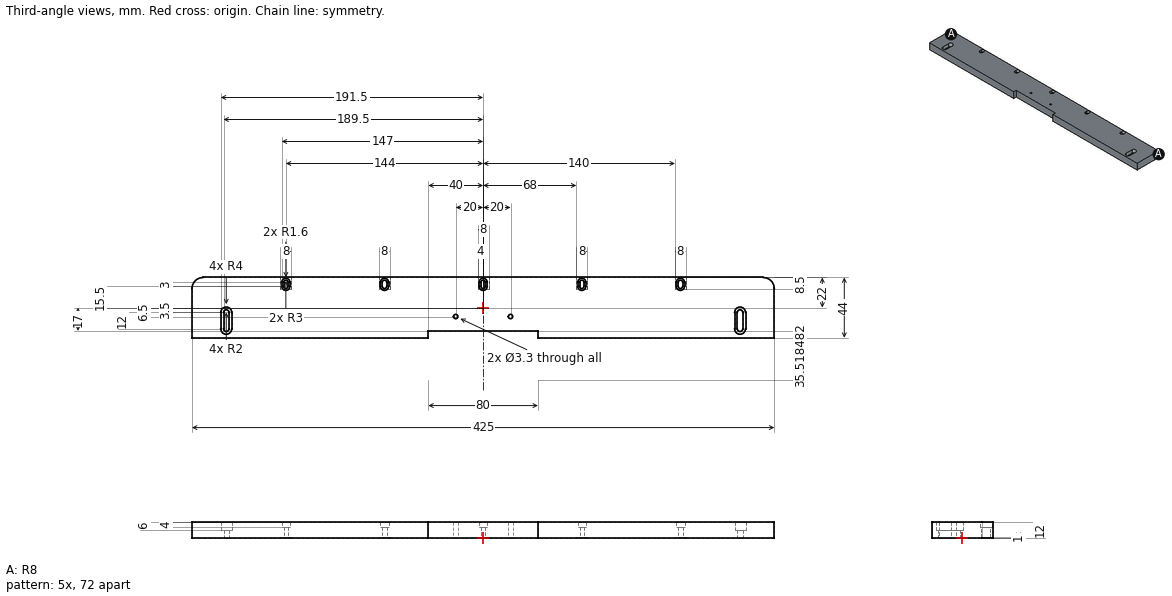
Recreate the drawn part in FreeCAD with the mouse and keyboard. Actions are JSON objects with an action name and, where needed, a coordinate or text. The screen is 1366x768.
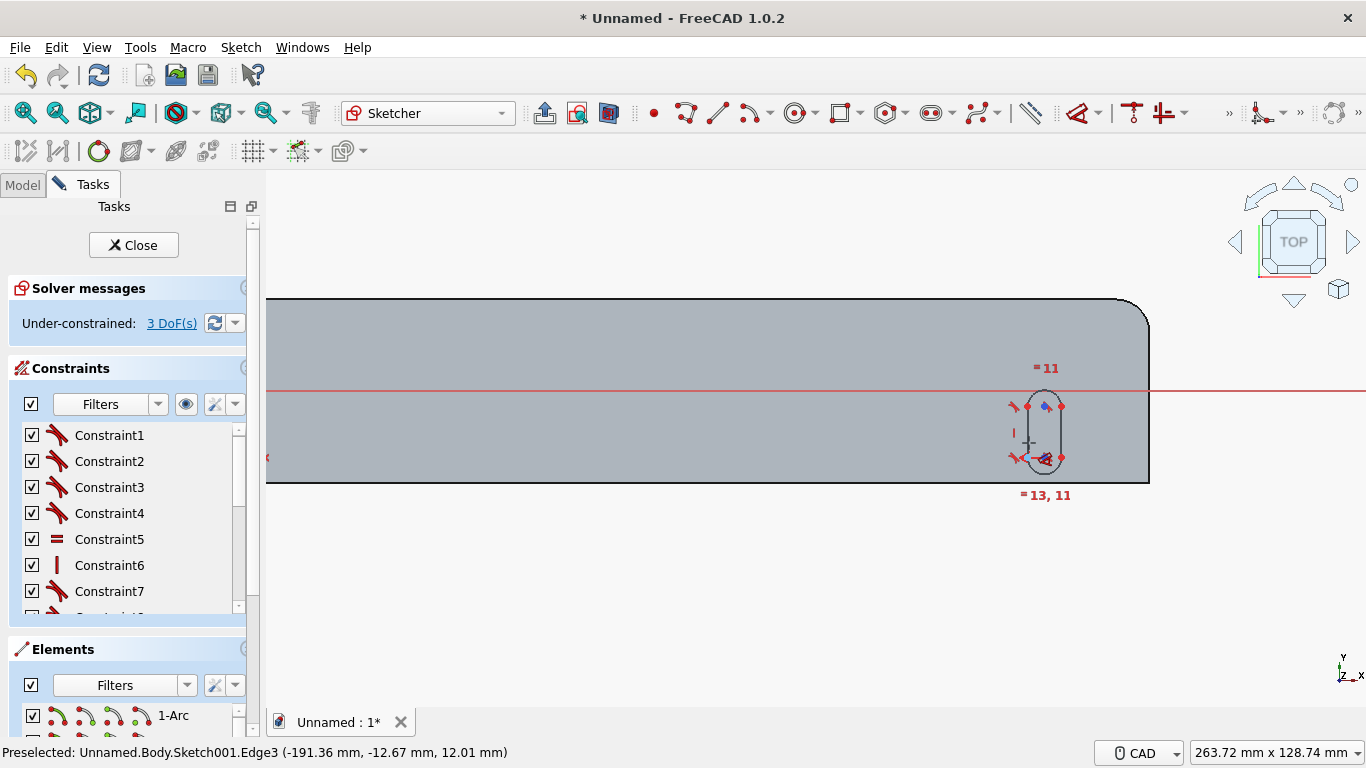
{"action": "left_click", "coordinate": [1028, 443]}
{"action": "left_click", "coordinate": [994, 432]}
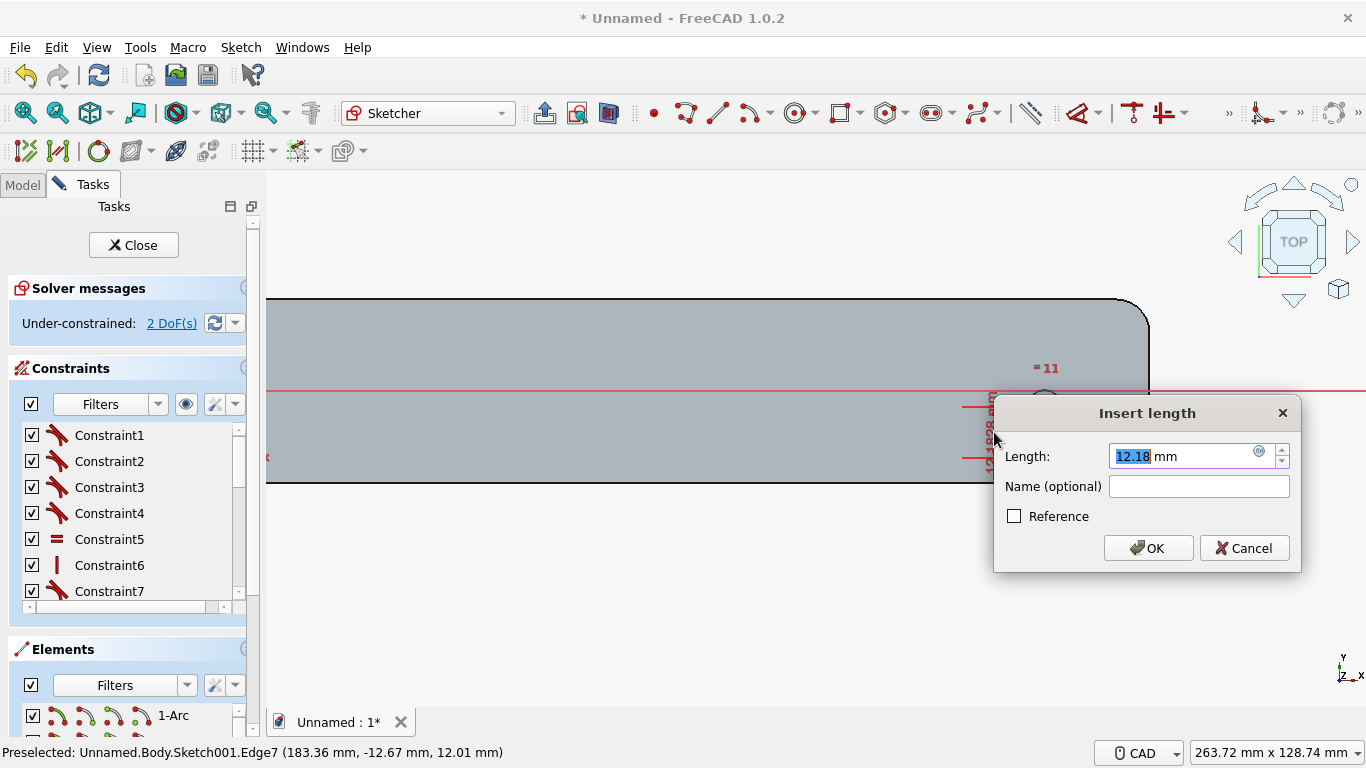
{"action": "type", "text": "12"}
{"action": "key", "text": "Return"}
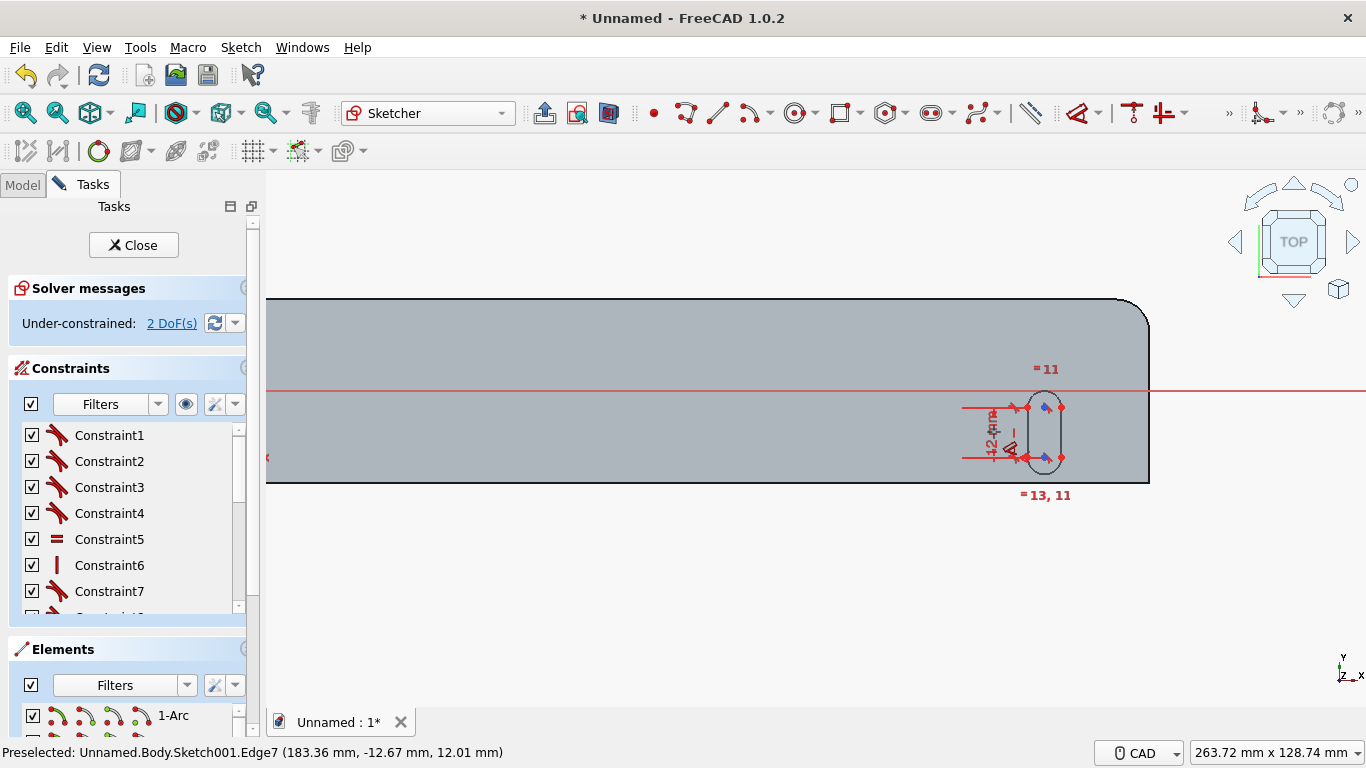
{"action": "scroll", "coordinate": [1029, 443], "scroll_direction": "down", "scroll_amount": 5}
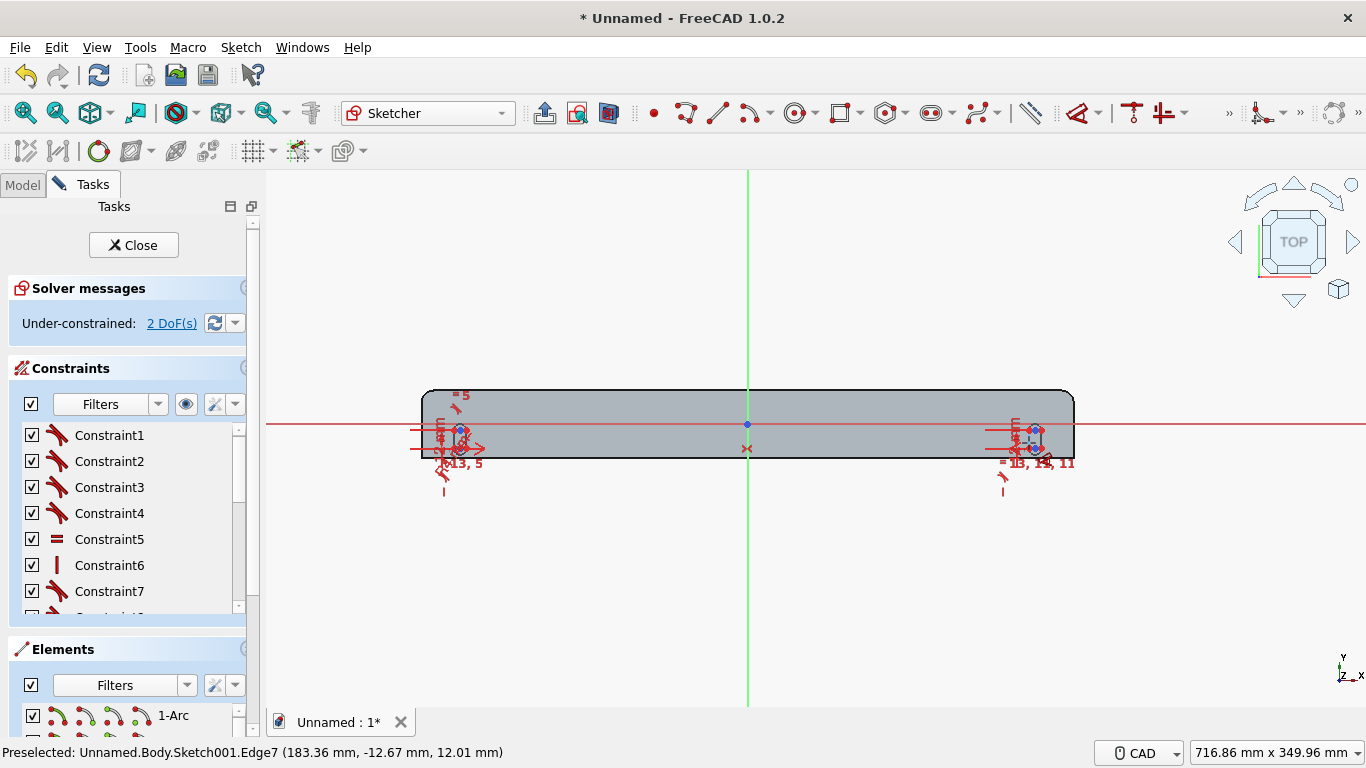
{"action": "scroll", "coordinate": [466, 430], "scroll_direction": "up", "scroll_amount": 11}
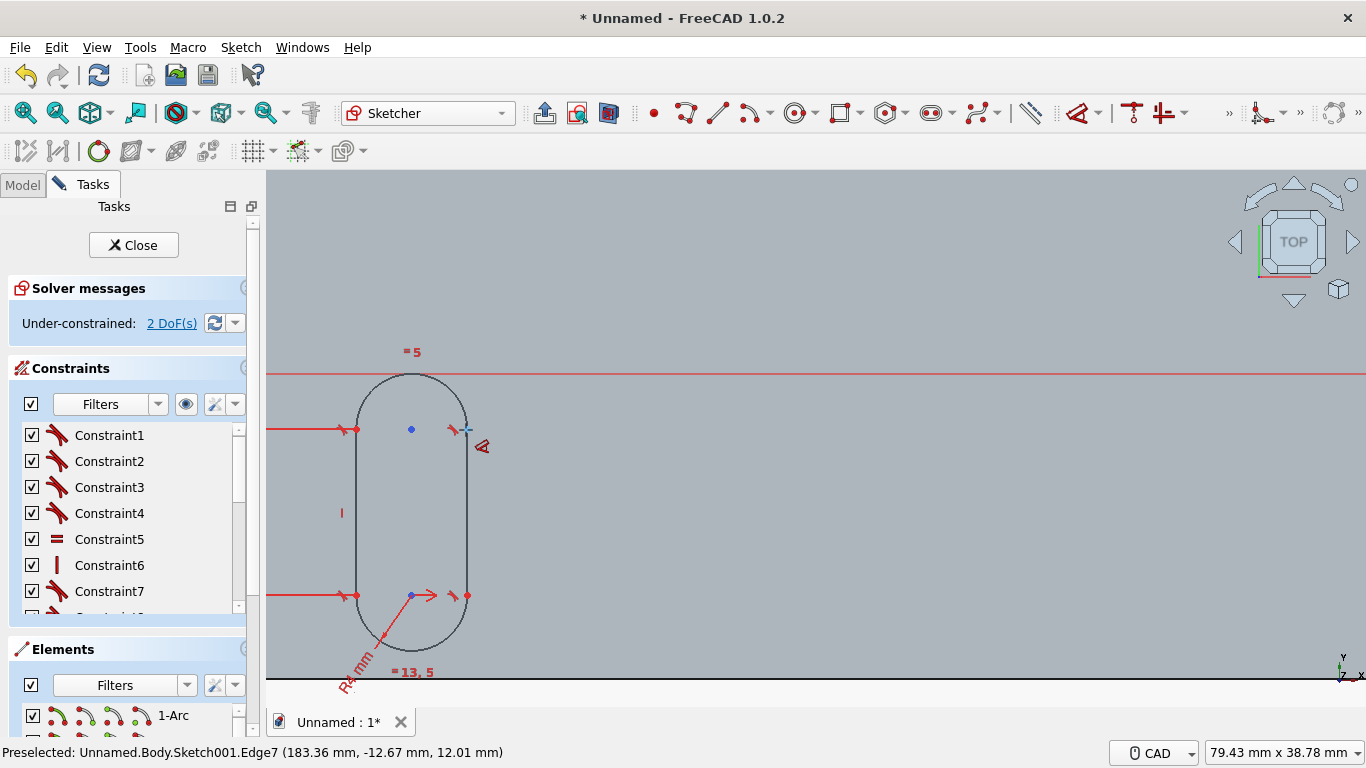
{"action": "left_click", "coordinate": [467, 429]}
{"action": "left_click", "coordinate": [433, 402]}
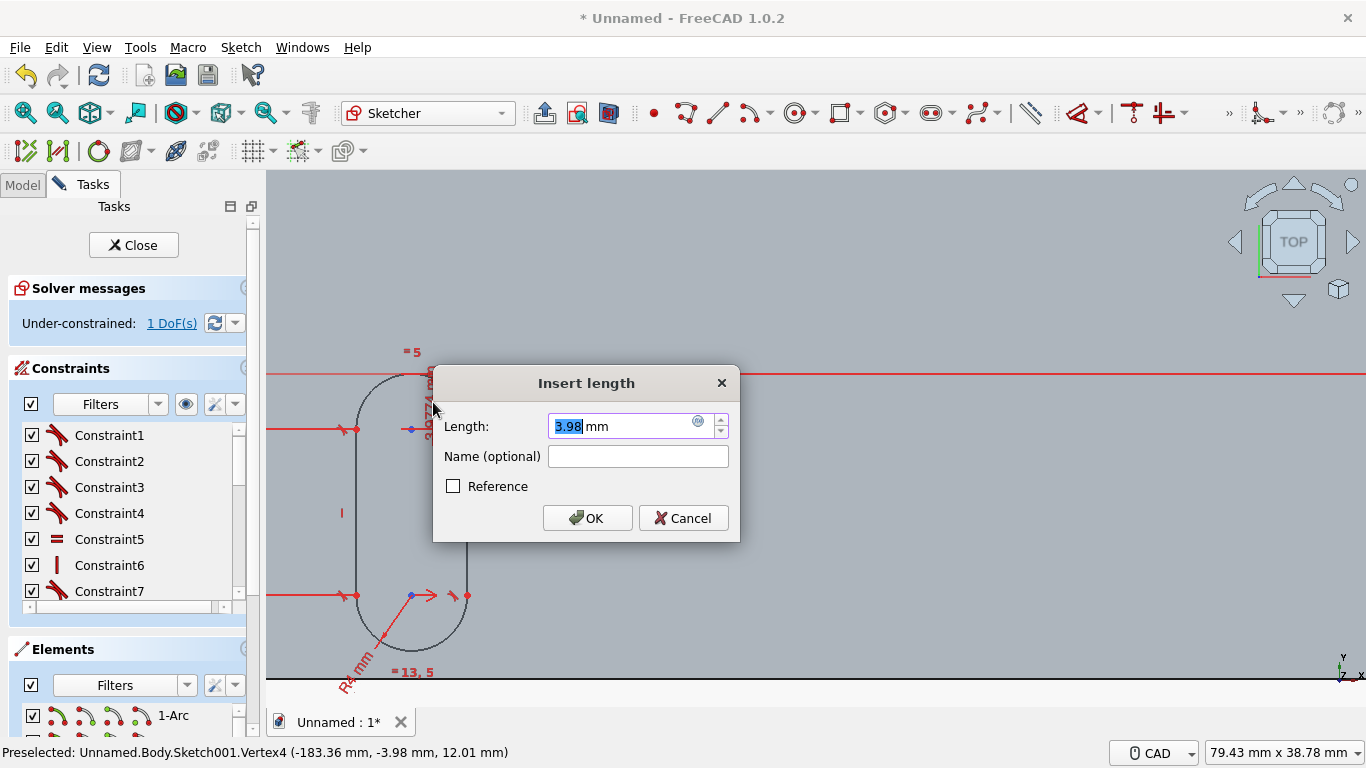
{"action": "type", "text": "3.5"}
{"action": "key", "text": "Return"}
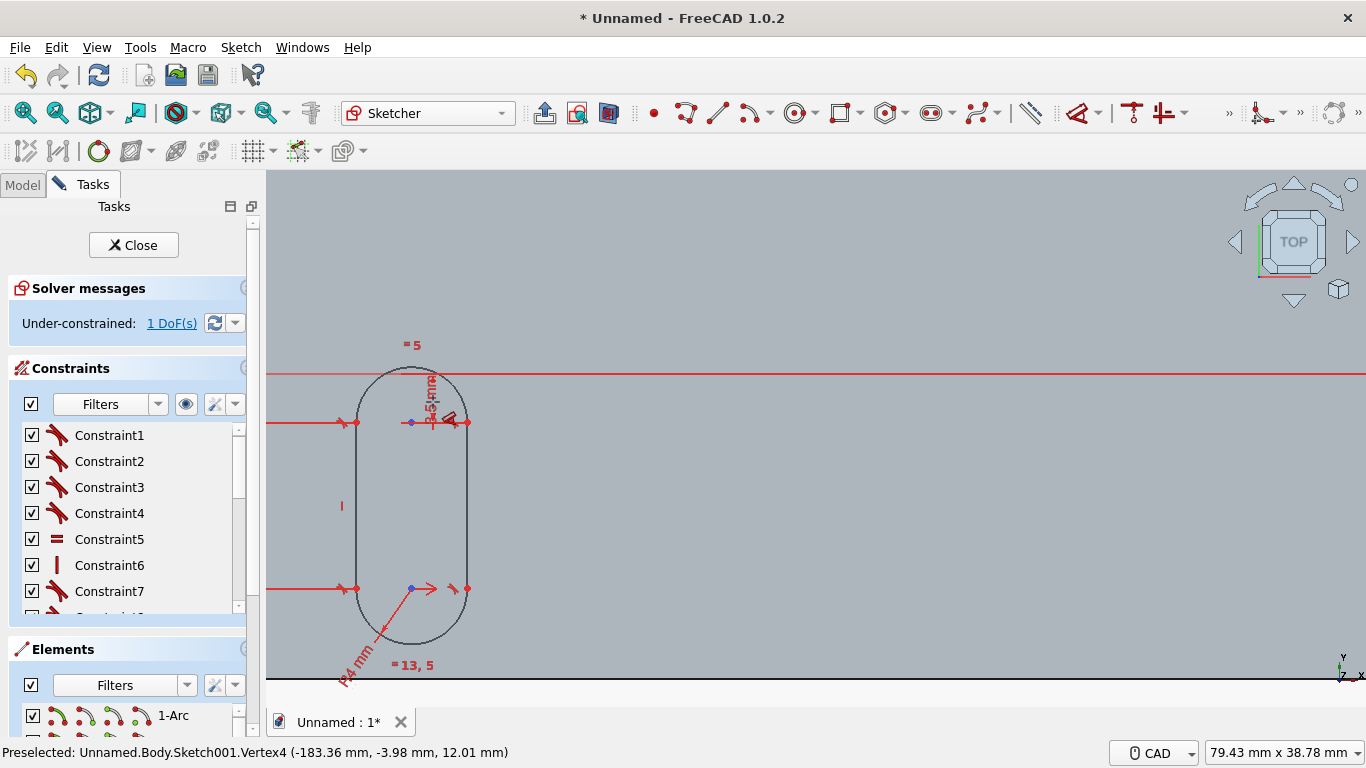
{"action": "scroll", "coordinate": [466, 430], "scroll_direction": "down", "scroll_amount": 11}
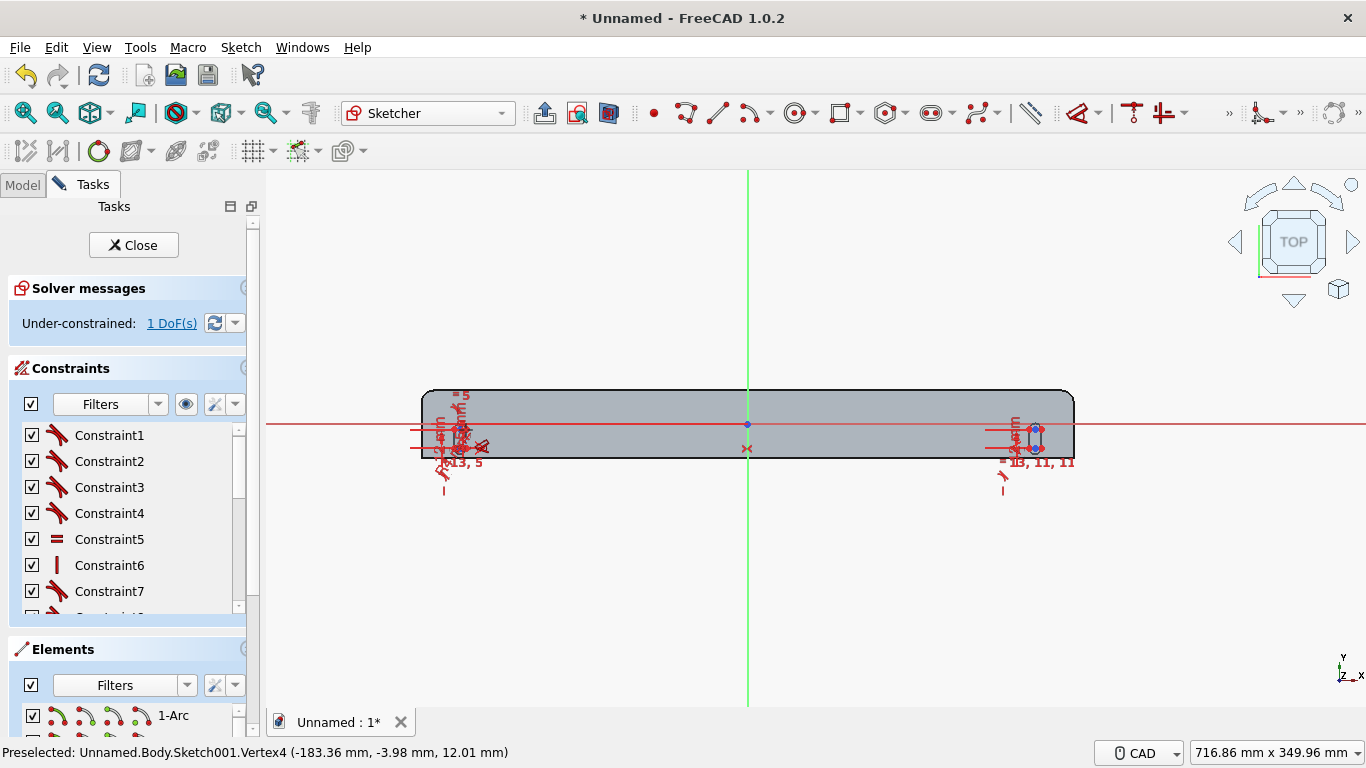
{"action": "scroll", "coordinate": [454, 448], "scroll_direction": "up", "scroll_amount": 4}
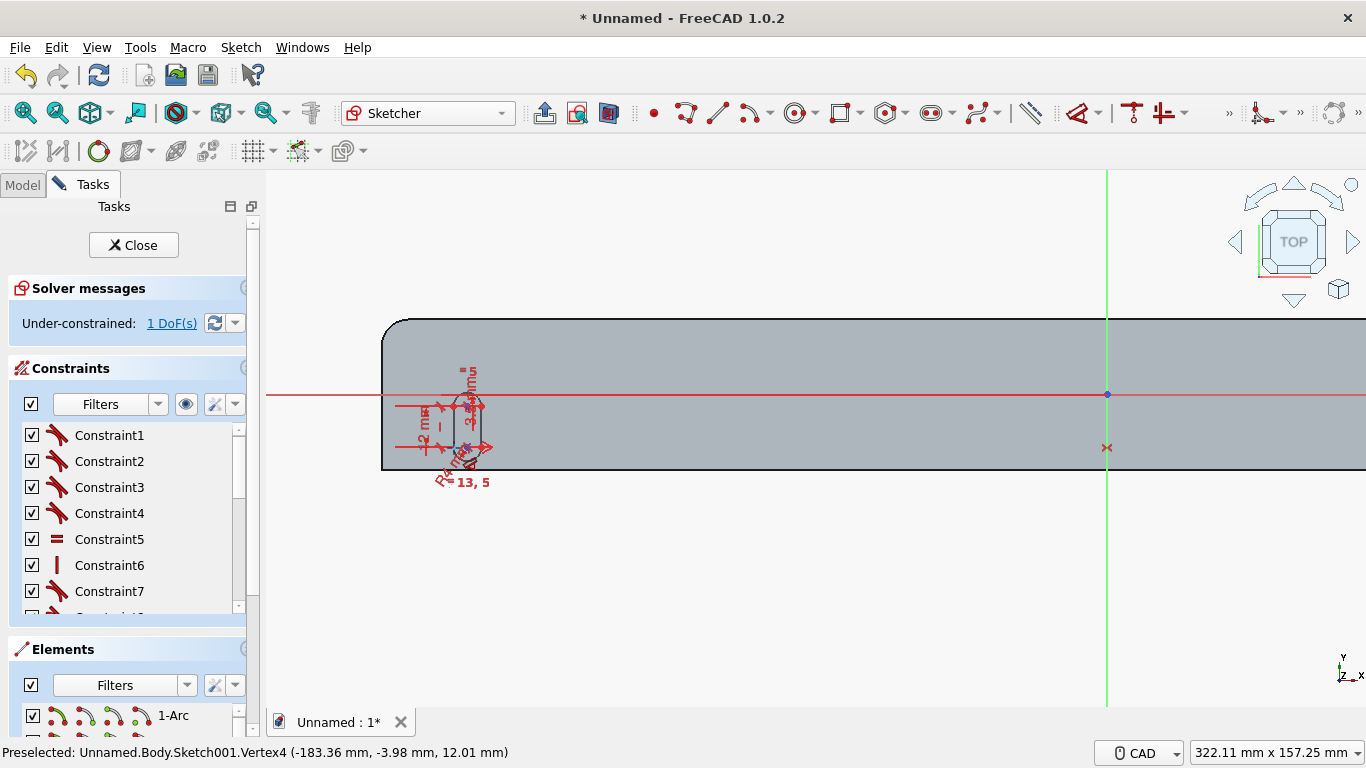
{"action": "left_click", "coordinate": [454, 447]}
{"action": "left_click", "coordinate": [781, 361]}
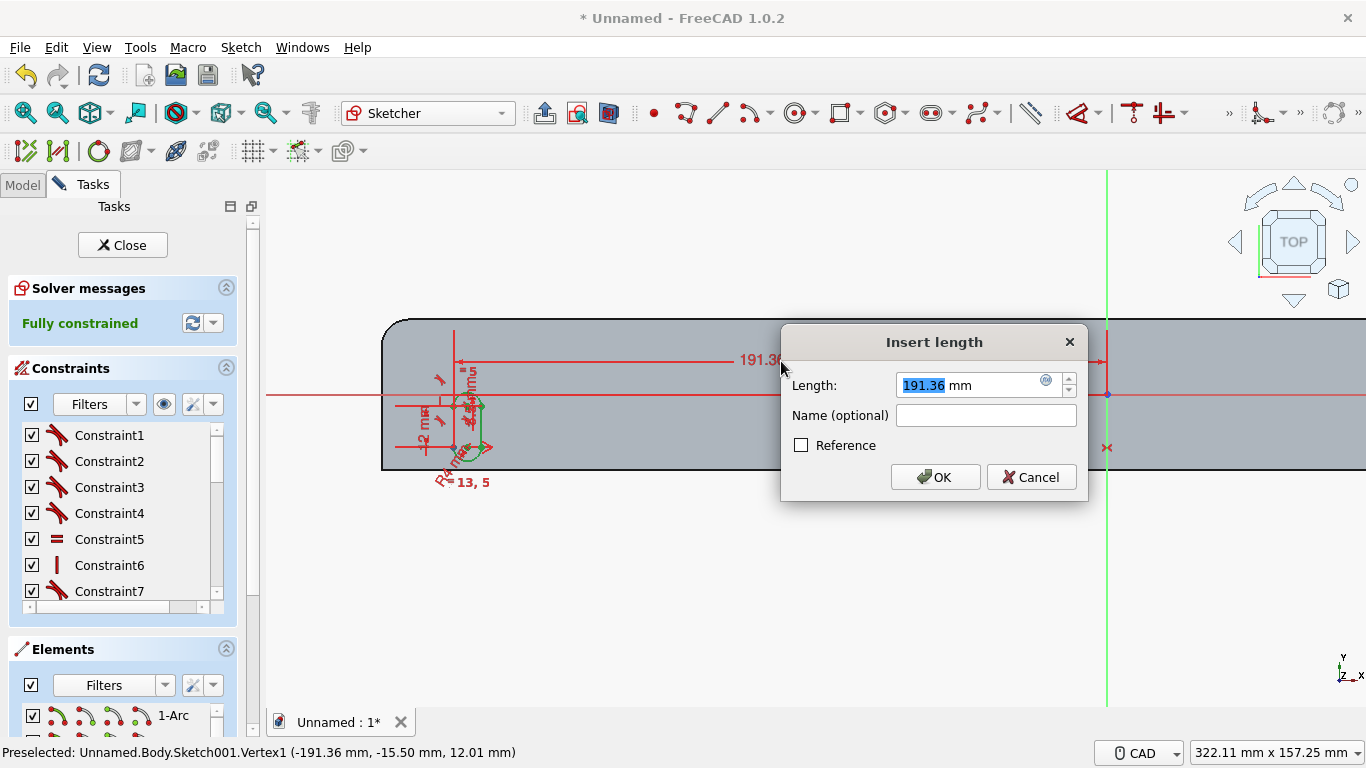
{"action": "type", "text": "191.5"}
{"action": "key", "text": "Return"}
{"action": "key", "text": "Escape"}